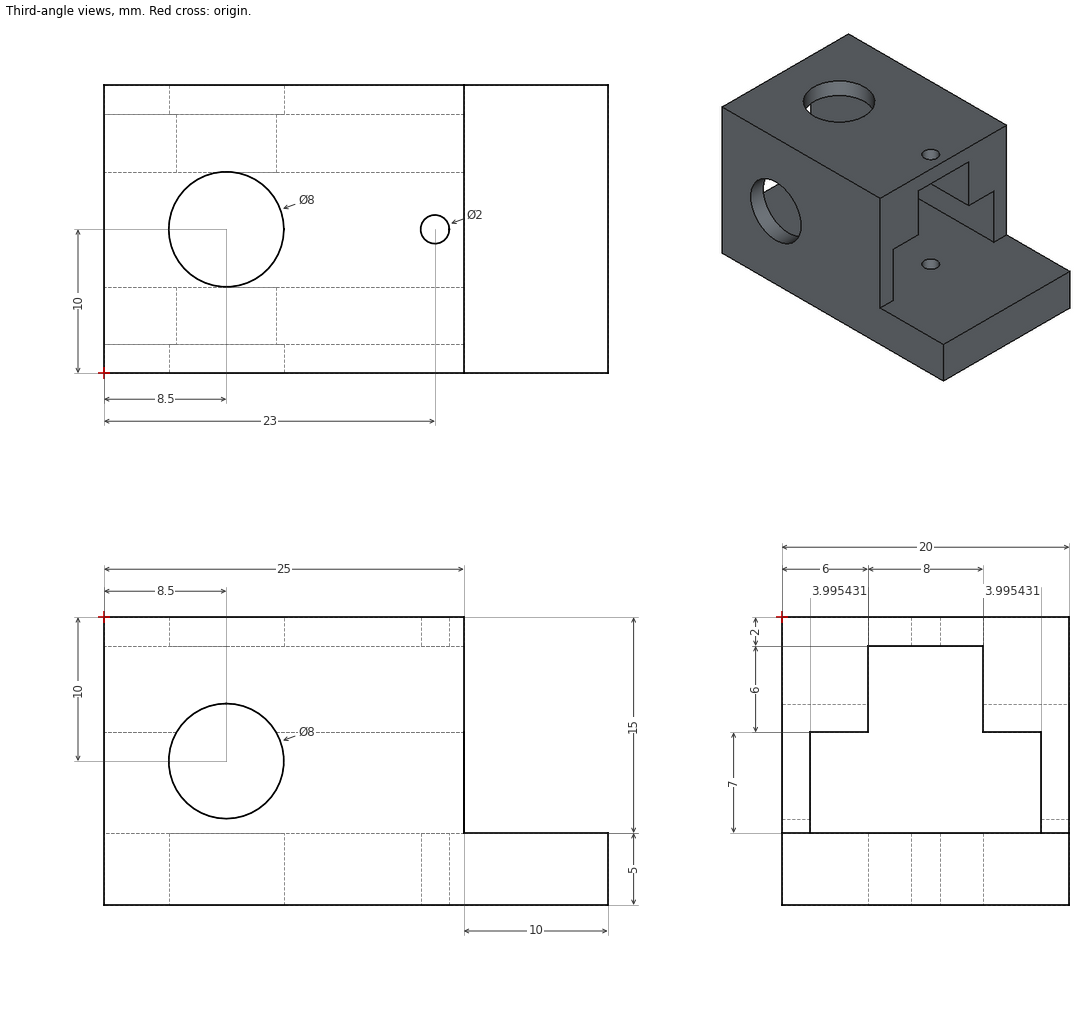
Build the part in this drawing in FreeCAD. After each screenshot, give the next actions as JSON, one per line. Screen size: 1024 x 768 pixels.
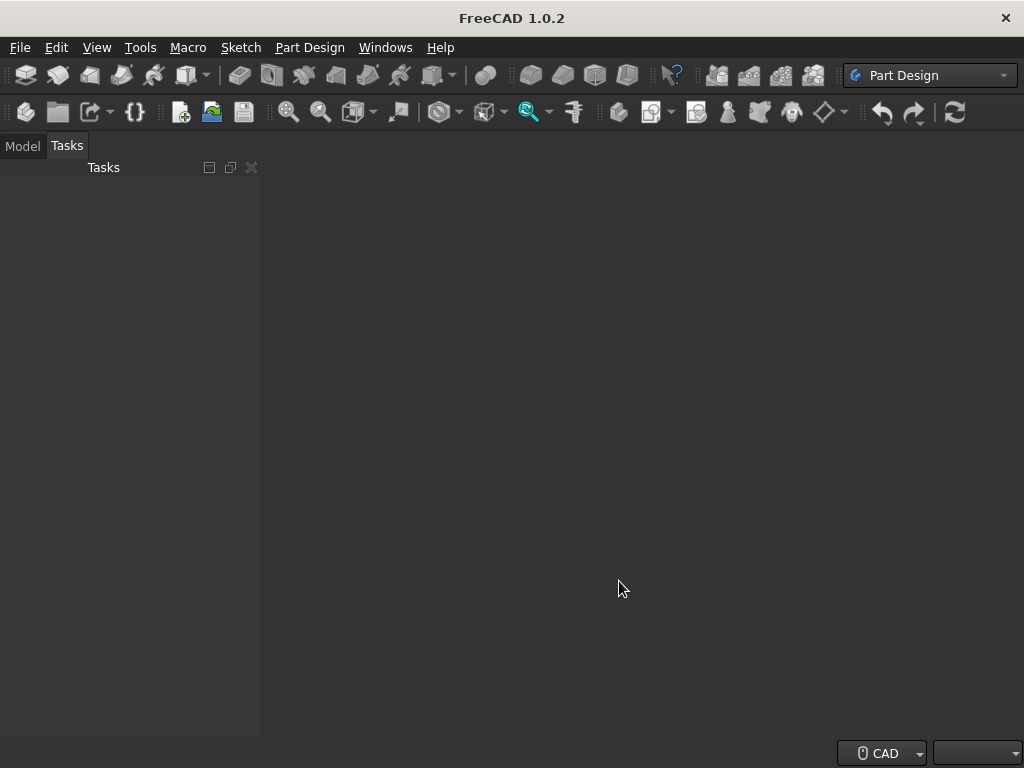
{"action": "left_click", "coordinate": [180, 112]}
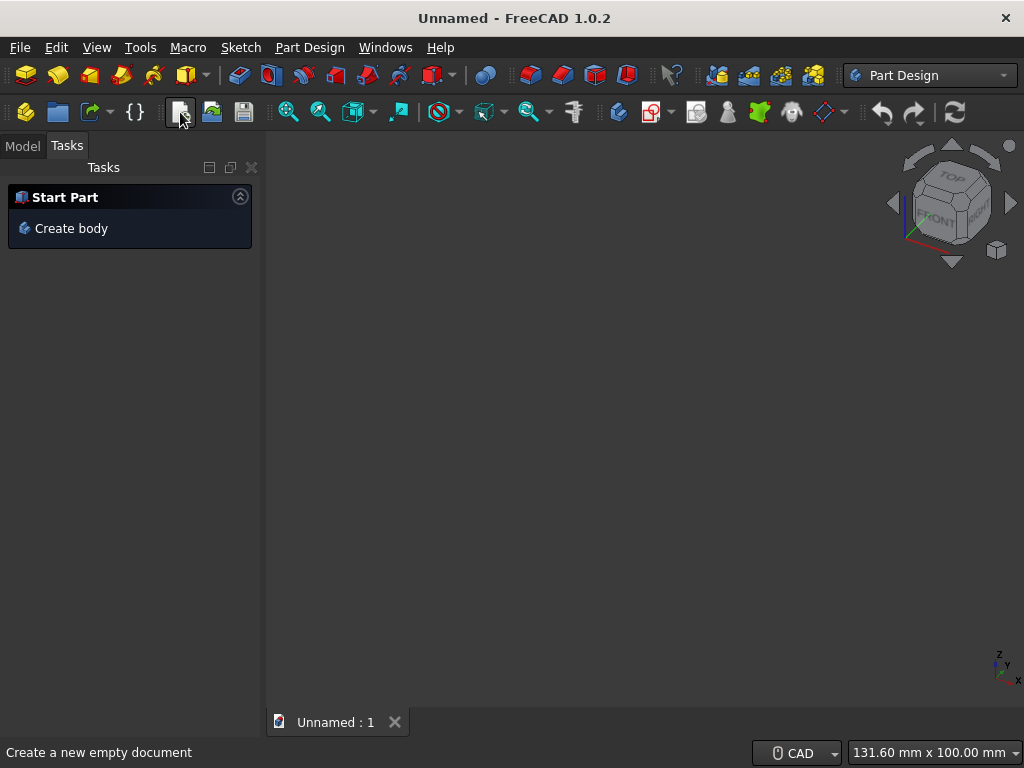
{"action": "left_click", "coordinate": [652, 112]}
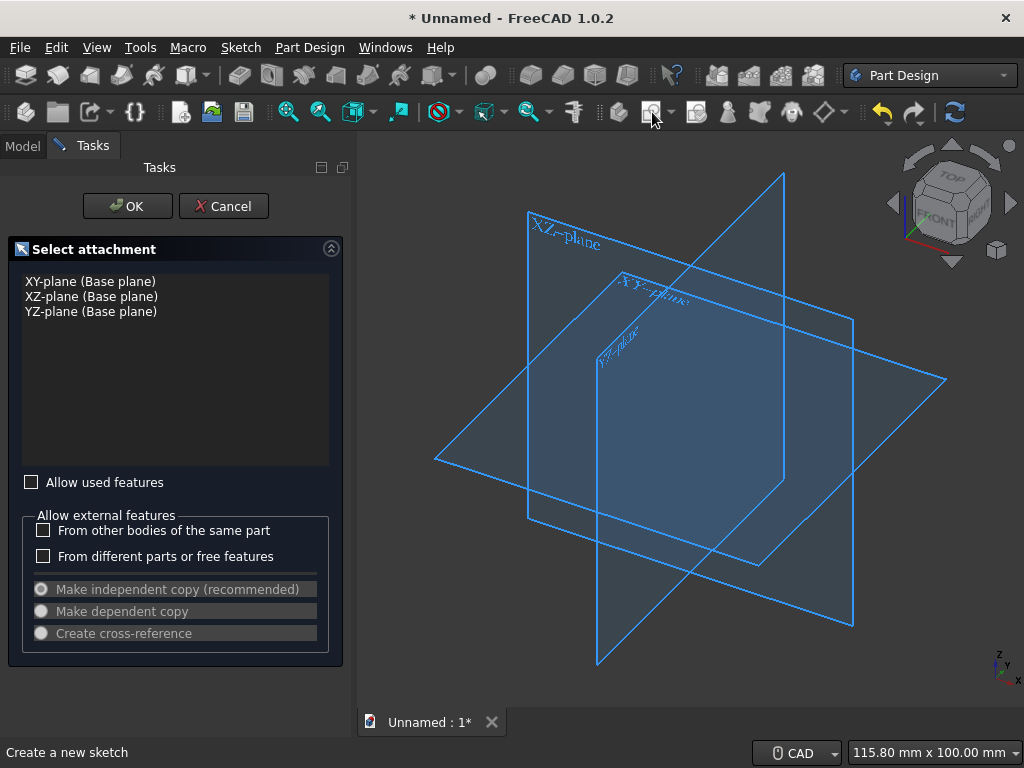
{"action": "left_click", "coordinate": [82, 296]}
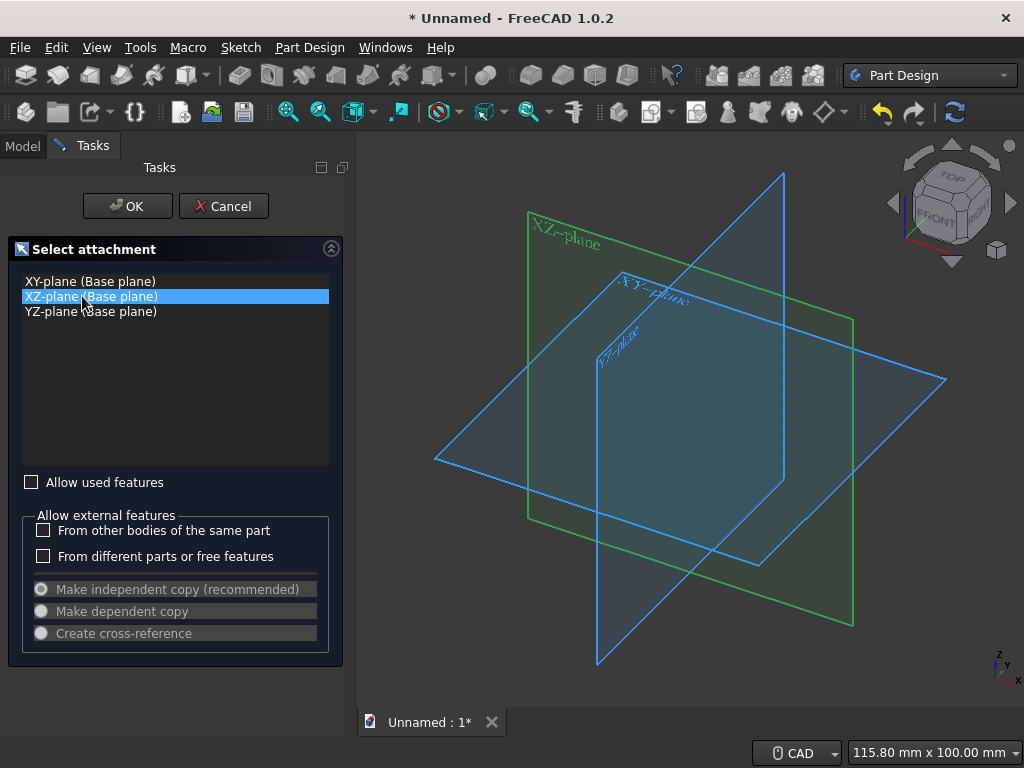
{"action": "left_click", "coordinate": [128, 206]}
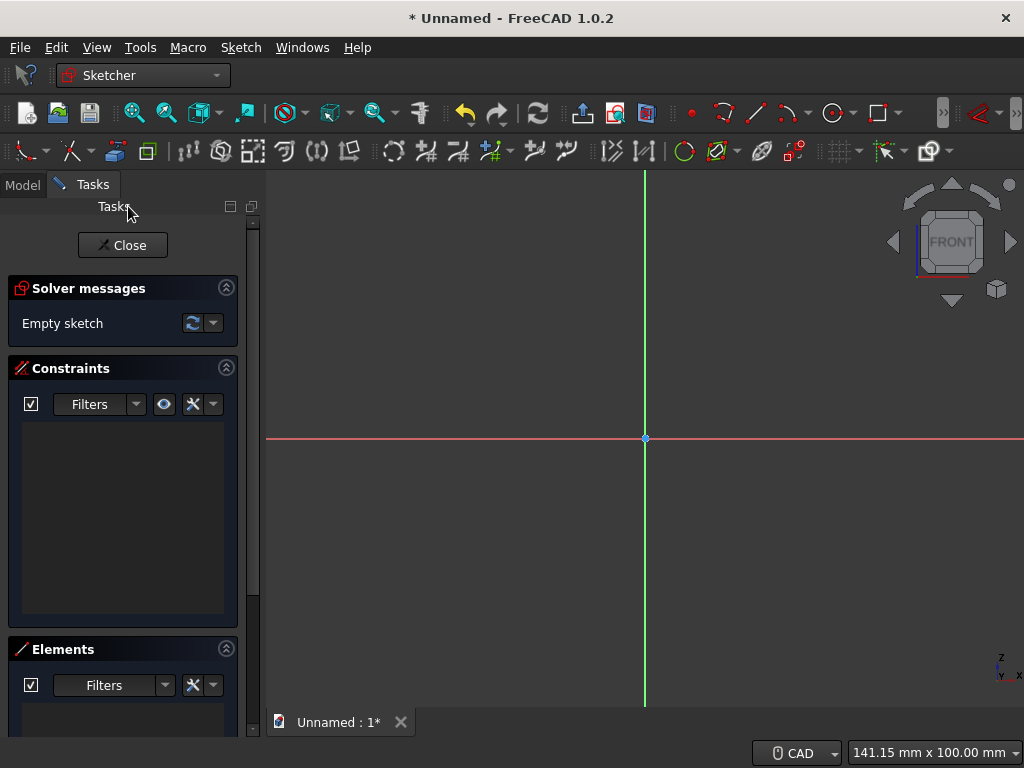
{"action": "scroll", "coordinate": [859, 536], "scroll_direction": "up", "scroll_amount": 4}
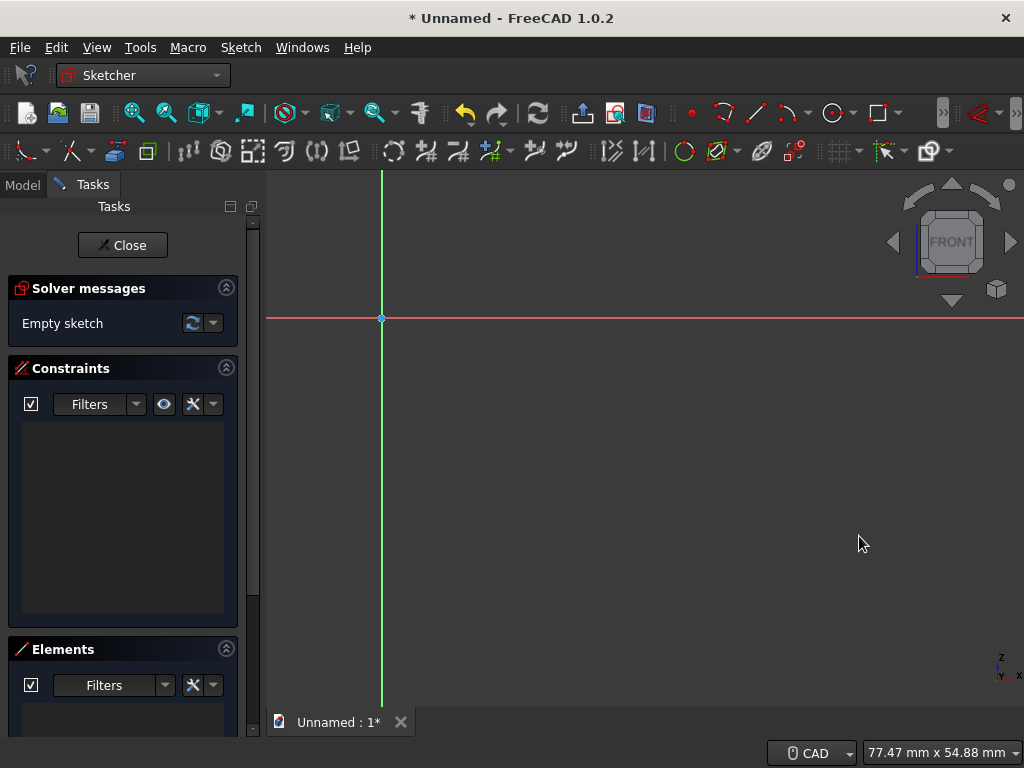
{"action": "left_click", "coordinate": [724, 114]}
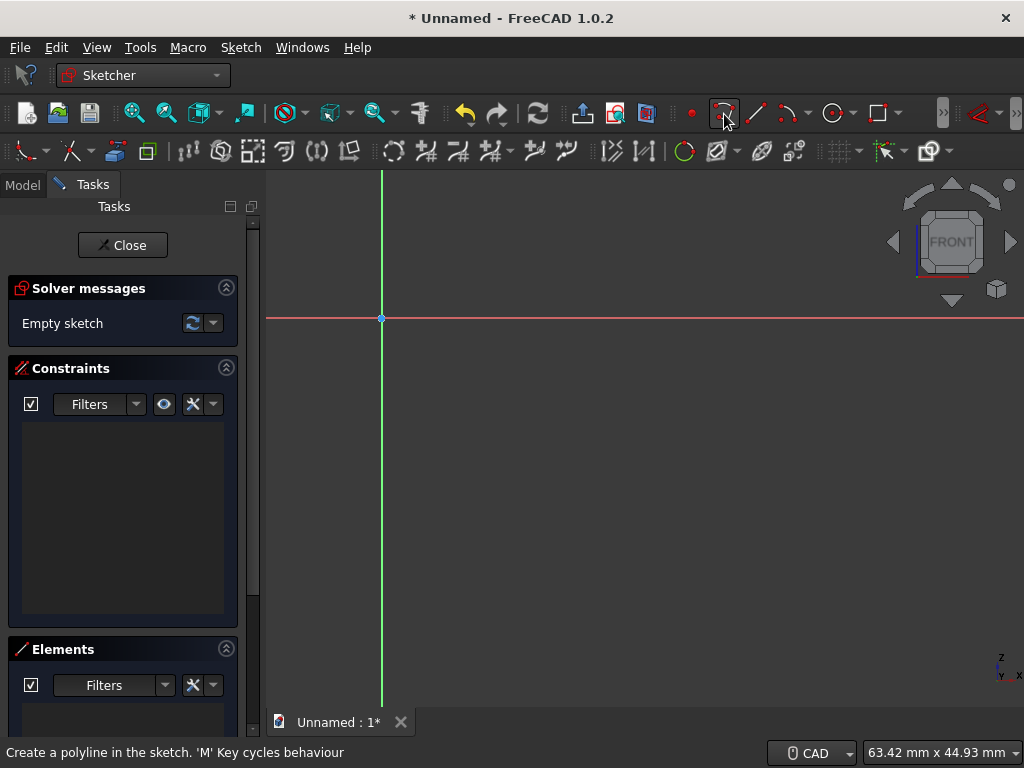
{"action": "left_click", "coordinate": [382, 318]}
{"action": "left_click", "coordinate": [681, 327]}
{"action": "left_click", "coordinate": [681, 497]}
{"action": "left_click", "coordinate": [800, 497]}
{"action": "left_click", "coordinate": [800, 557]}
{"action": "left_click", "coordinate": [391, 557]}
{"action": "left_click", "coordinate": [382, 318]}
{"action": "key", "text": "Escape"}
{"action": "key", "text": "Escape"}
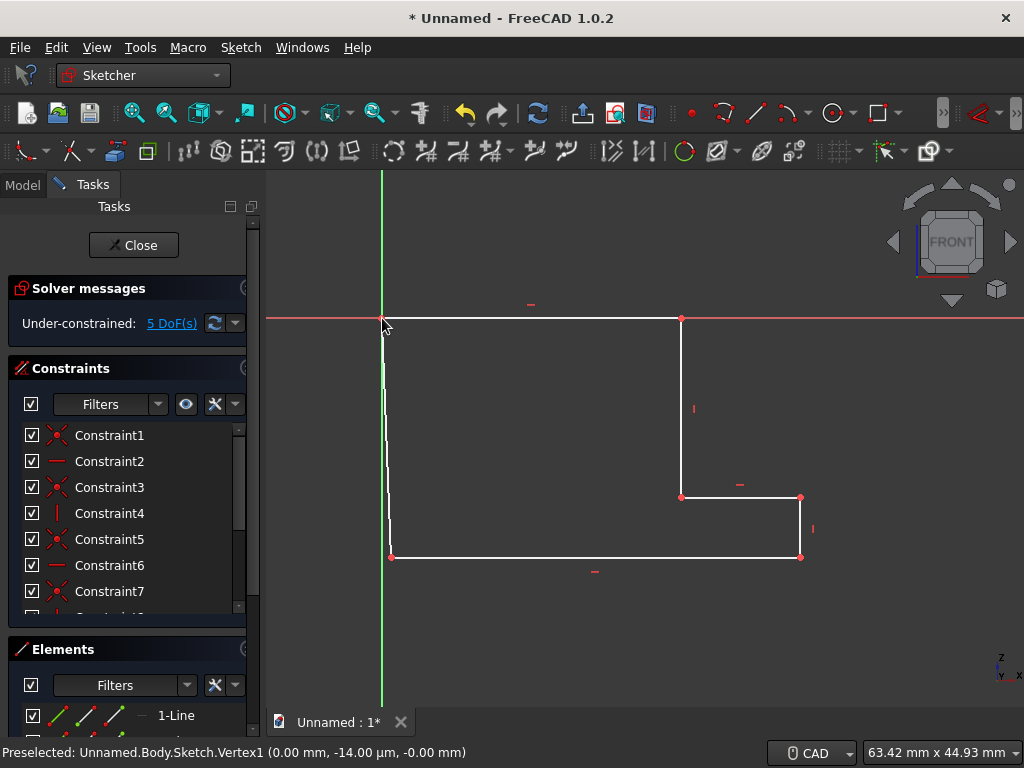
{"action": "left_click", "coordinate": [385, 390]}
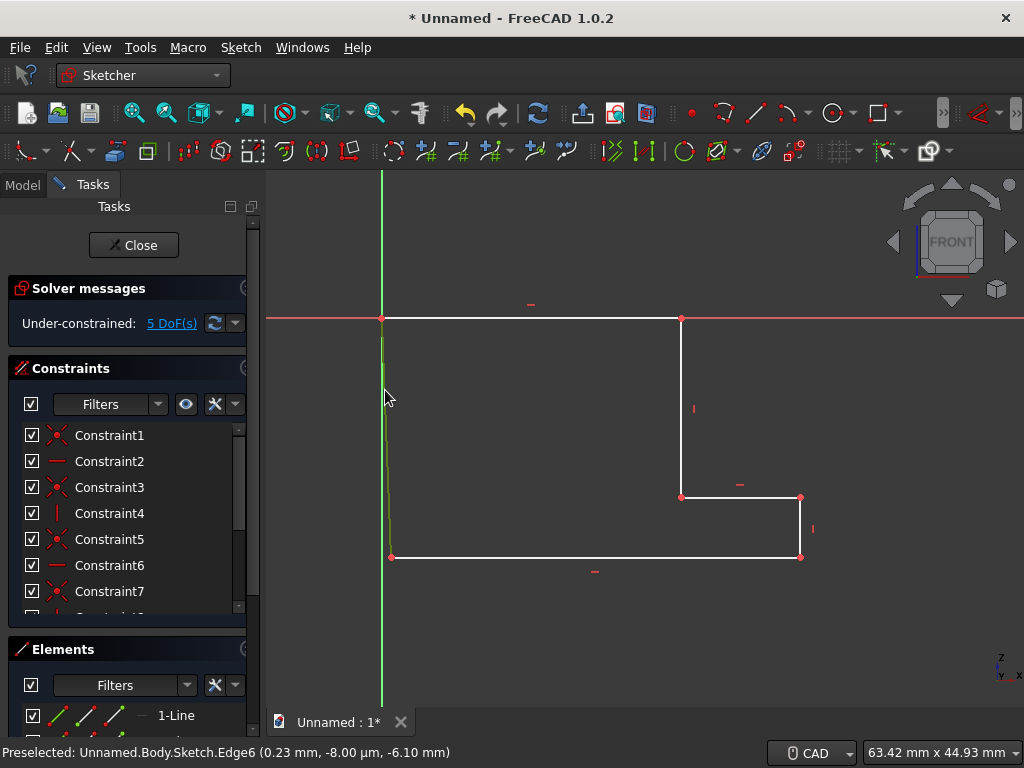
{"action": "key", "text": "v"}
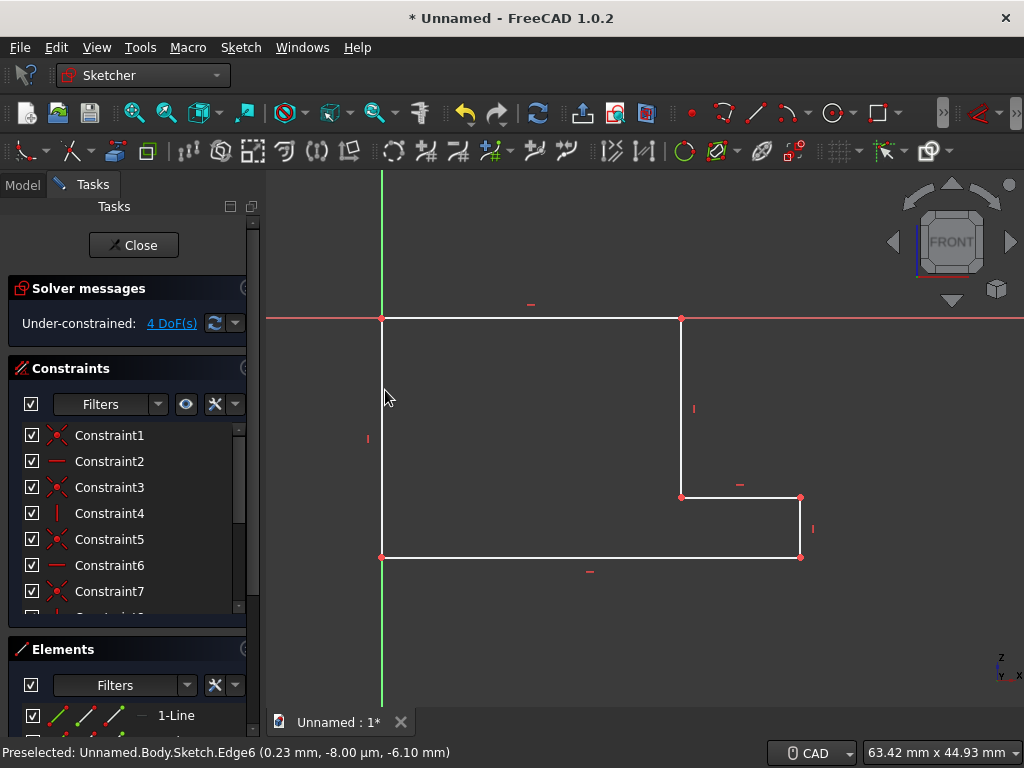
{"action": "left_click", "coordinate": [978, 114]}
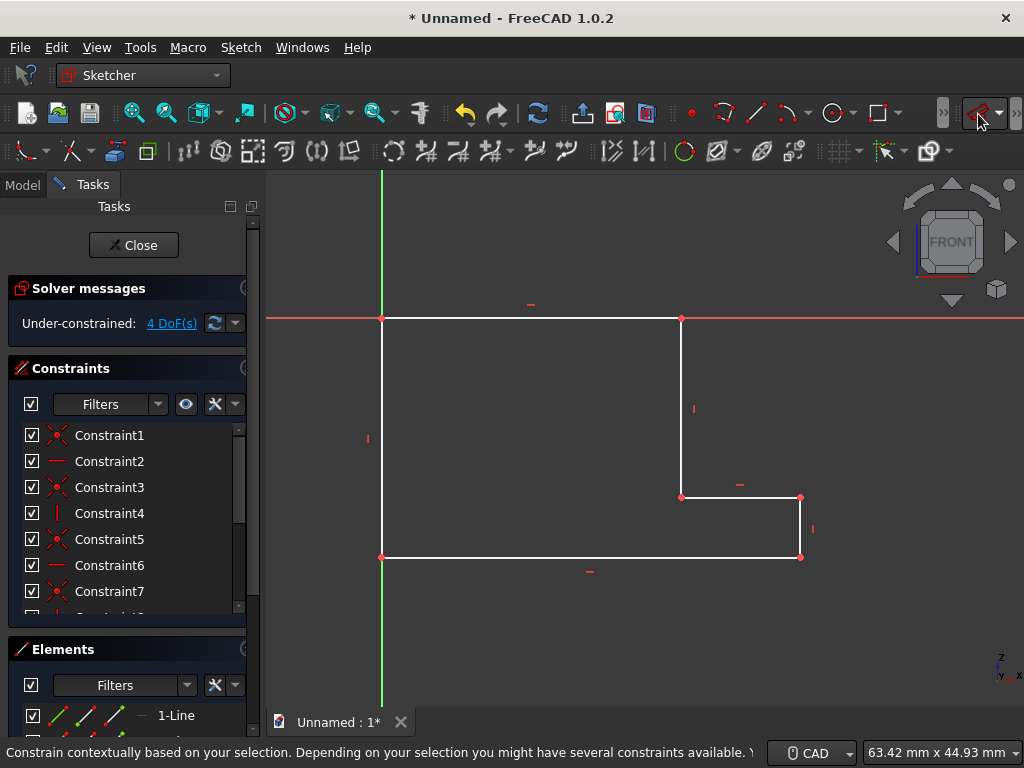
{"action": "left_click", "coordinate": [800, 516]}
{"action": "left_click", "coordinate": [834, 528]}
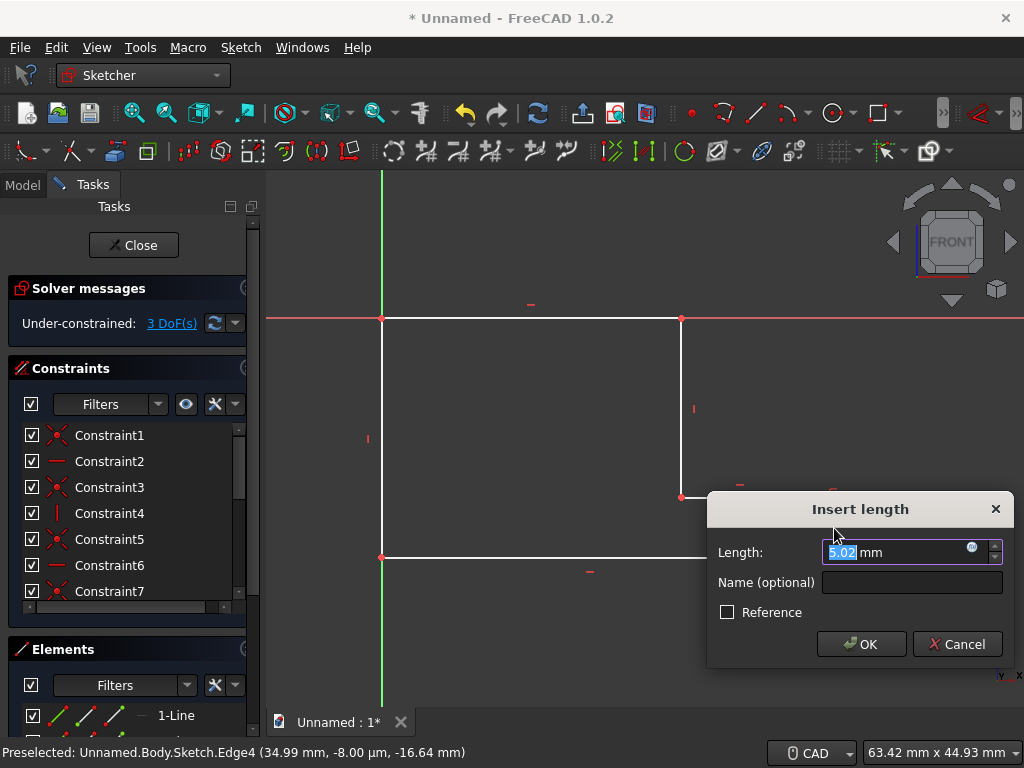
{"action": "type", "text": "5"}
{"action": "key", "text": "Return"}